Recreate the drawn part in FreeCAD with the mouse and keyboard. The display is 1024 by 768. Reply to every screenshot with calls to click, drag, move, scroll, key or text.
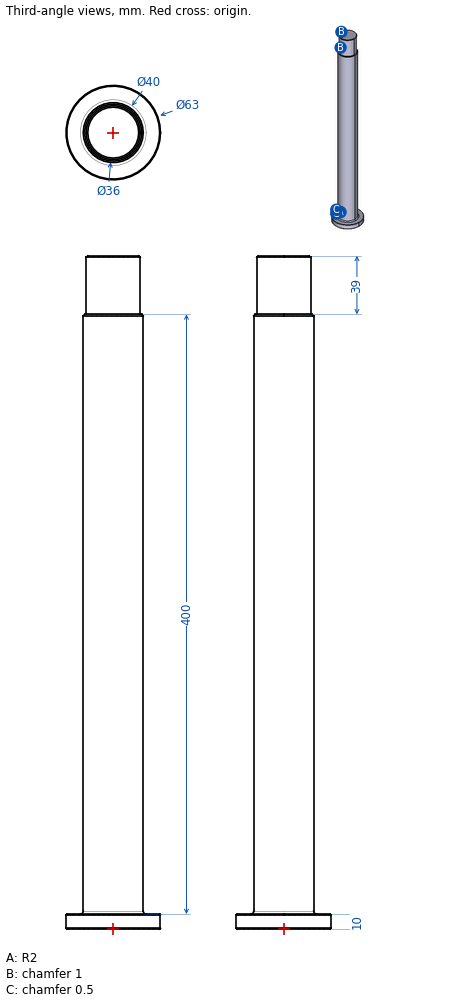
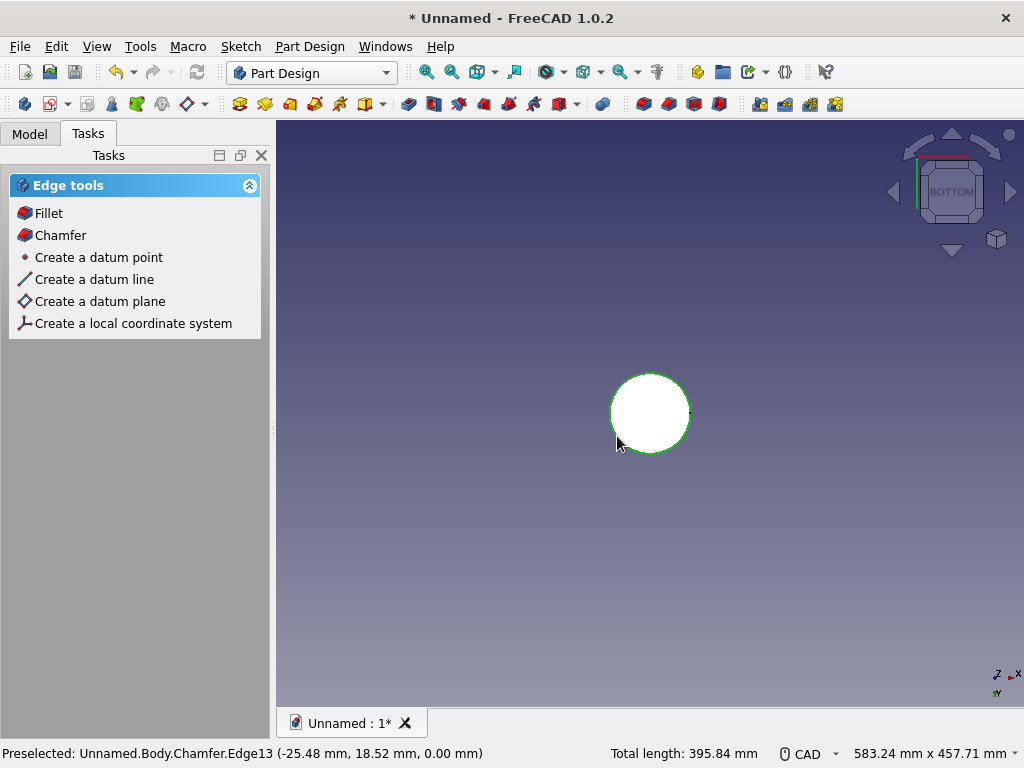
click(669, 104)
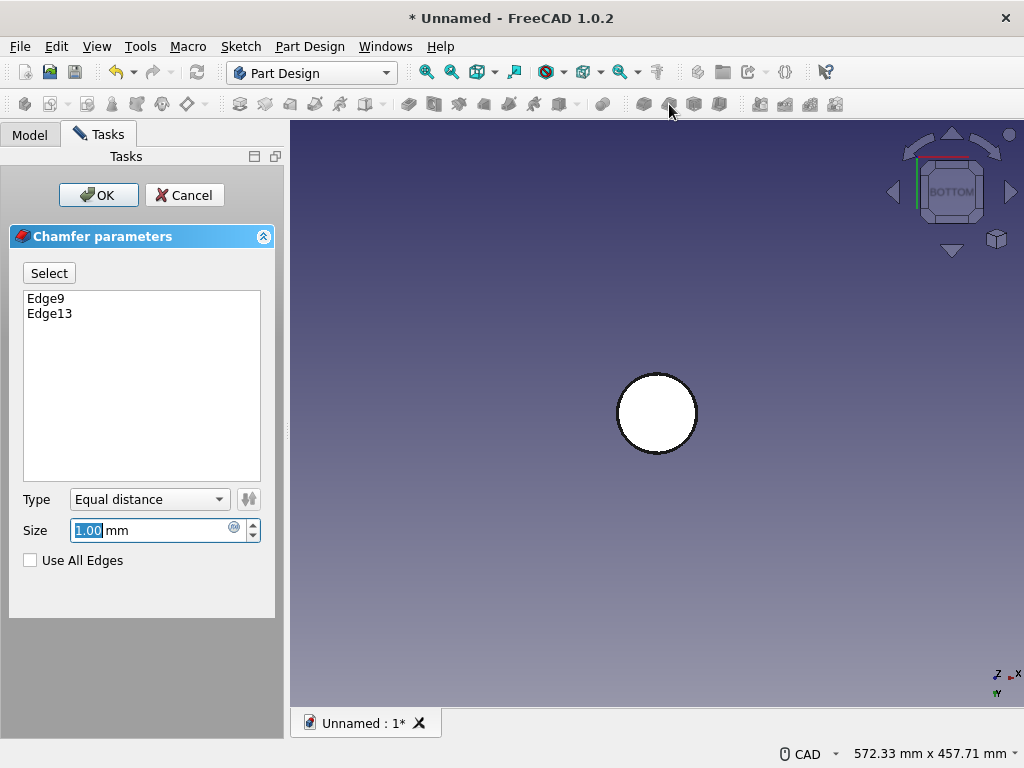
text(0.5)
key(Tab)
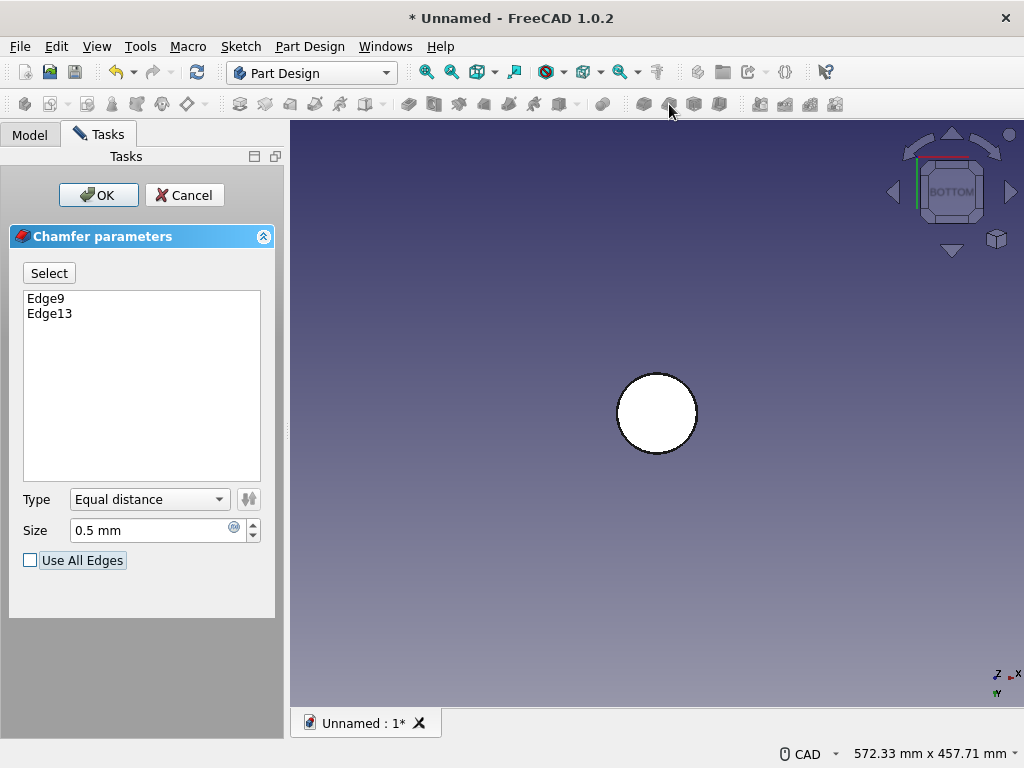
click(99, 195)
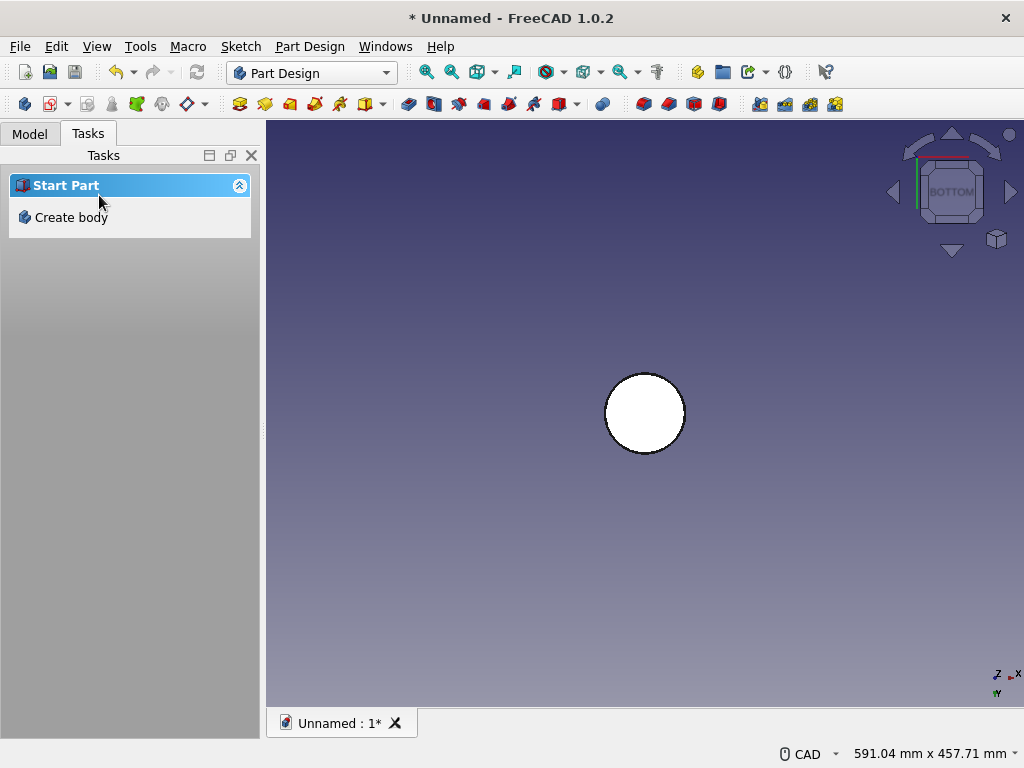
key(0)